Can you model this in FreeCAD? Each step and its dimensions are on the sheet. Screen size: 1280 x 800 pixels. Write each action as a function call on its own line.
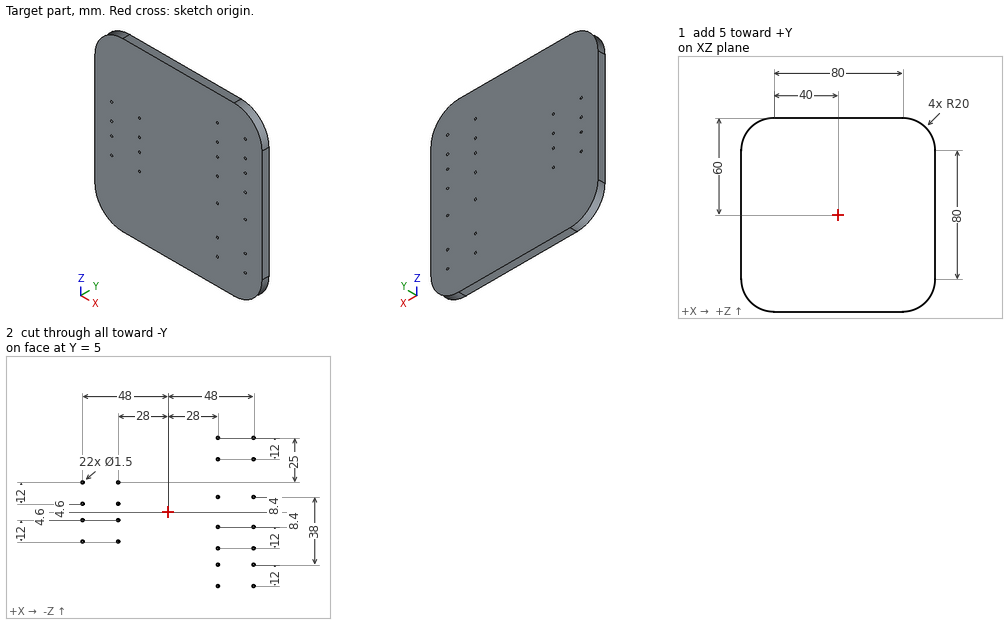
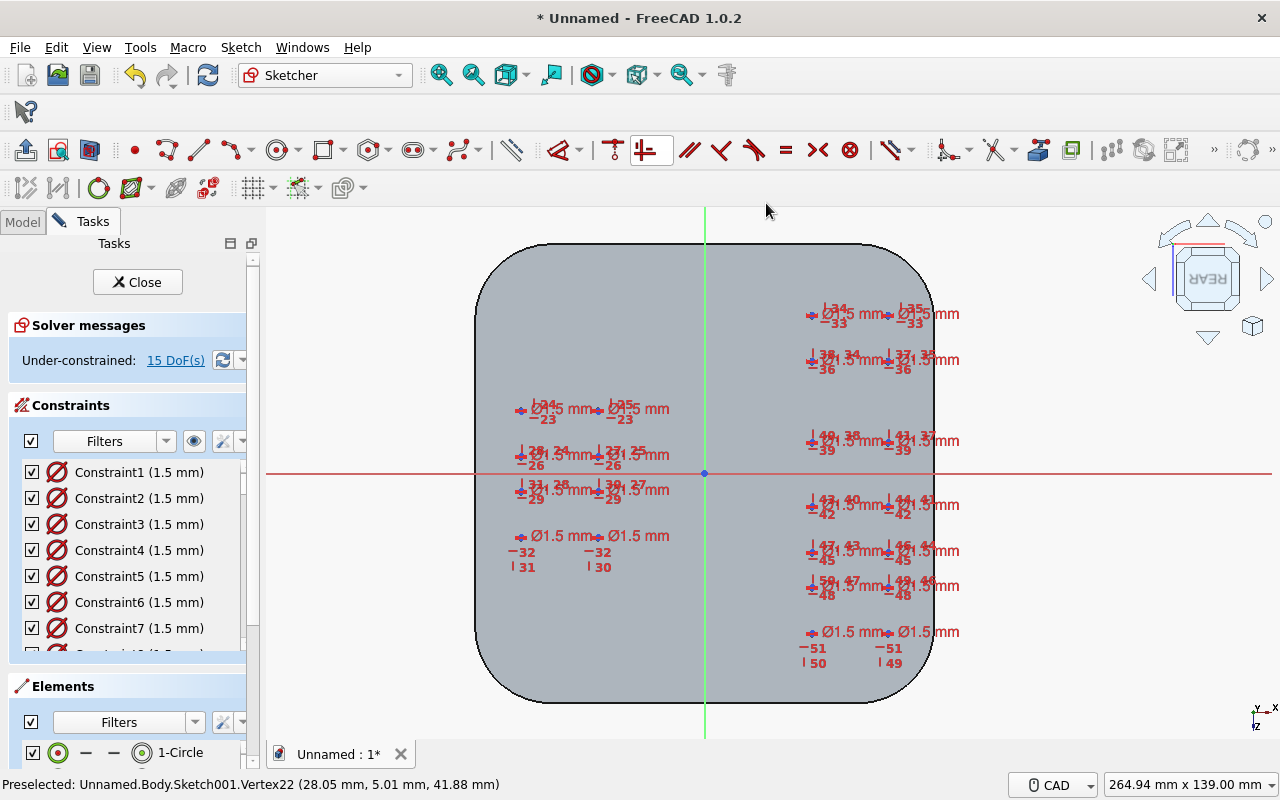
click(558, 150)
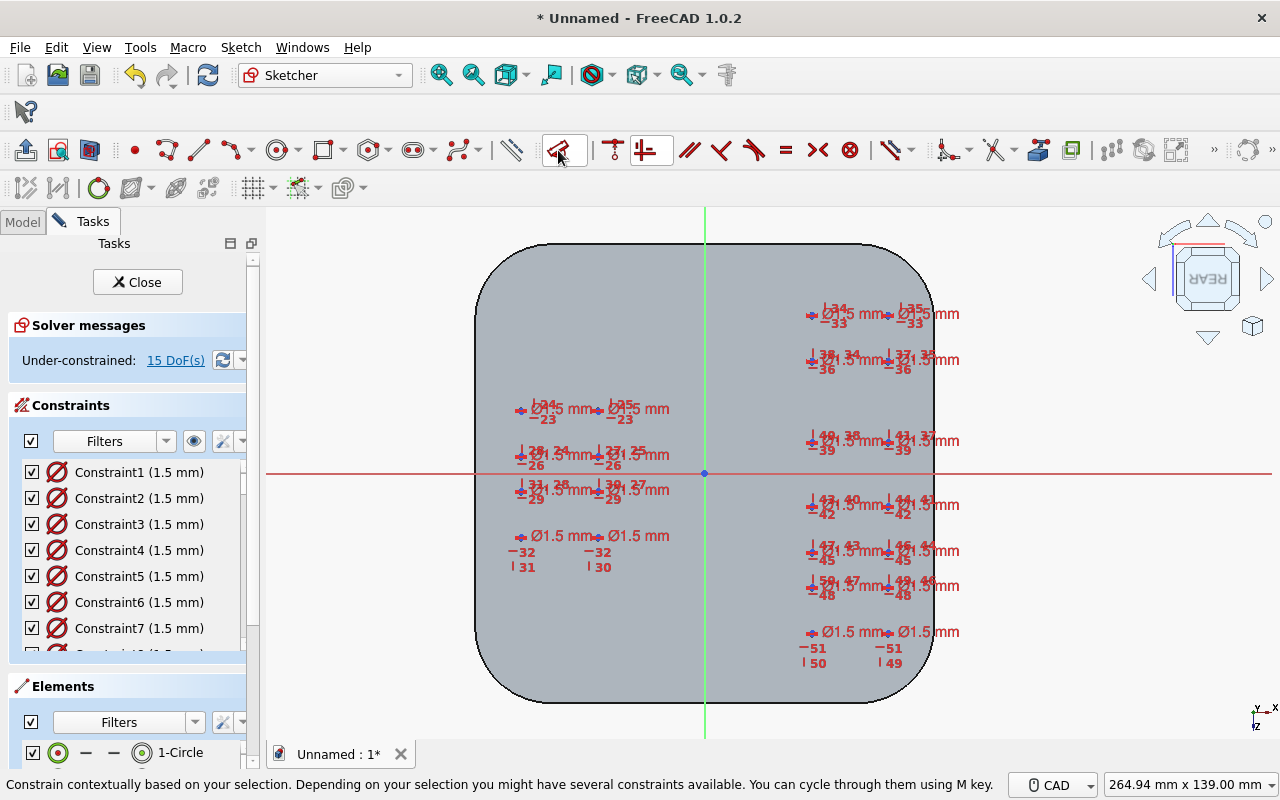
click(521, 411)
click(613, 377)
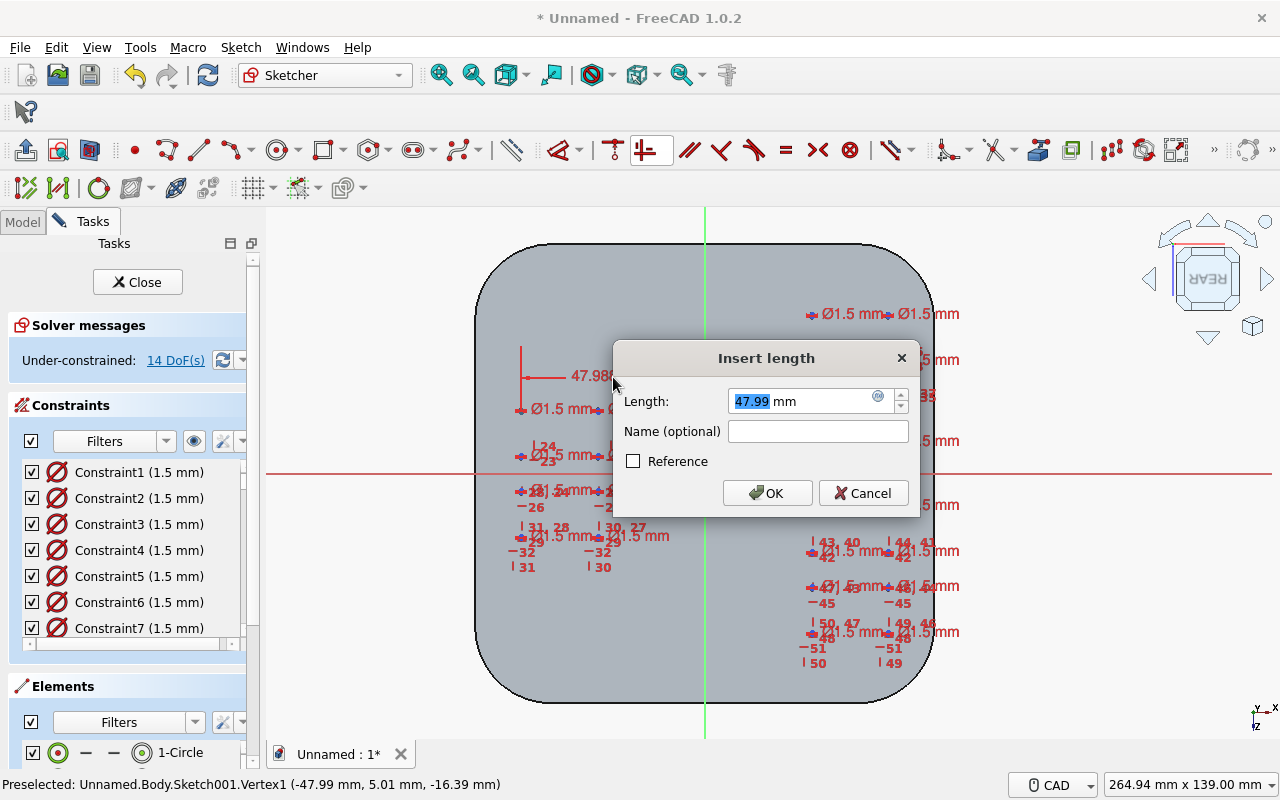
text(48)
key(Return)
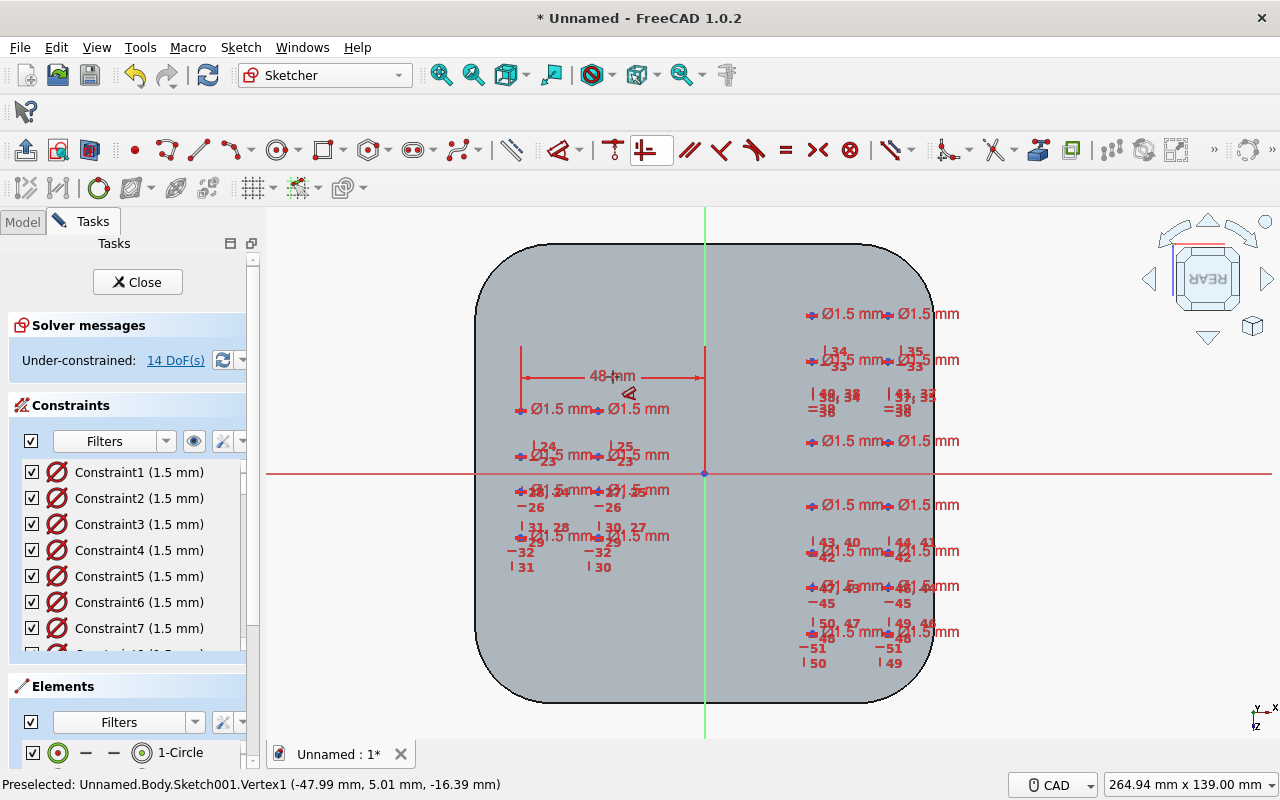
click(598, 411)
click(689, 377)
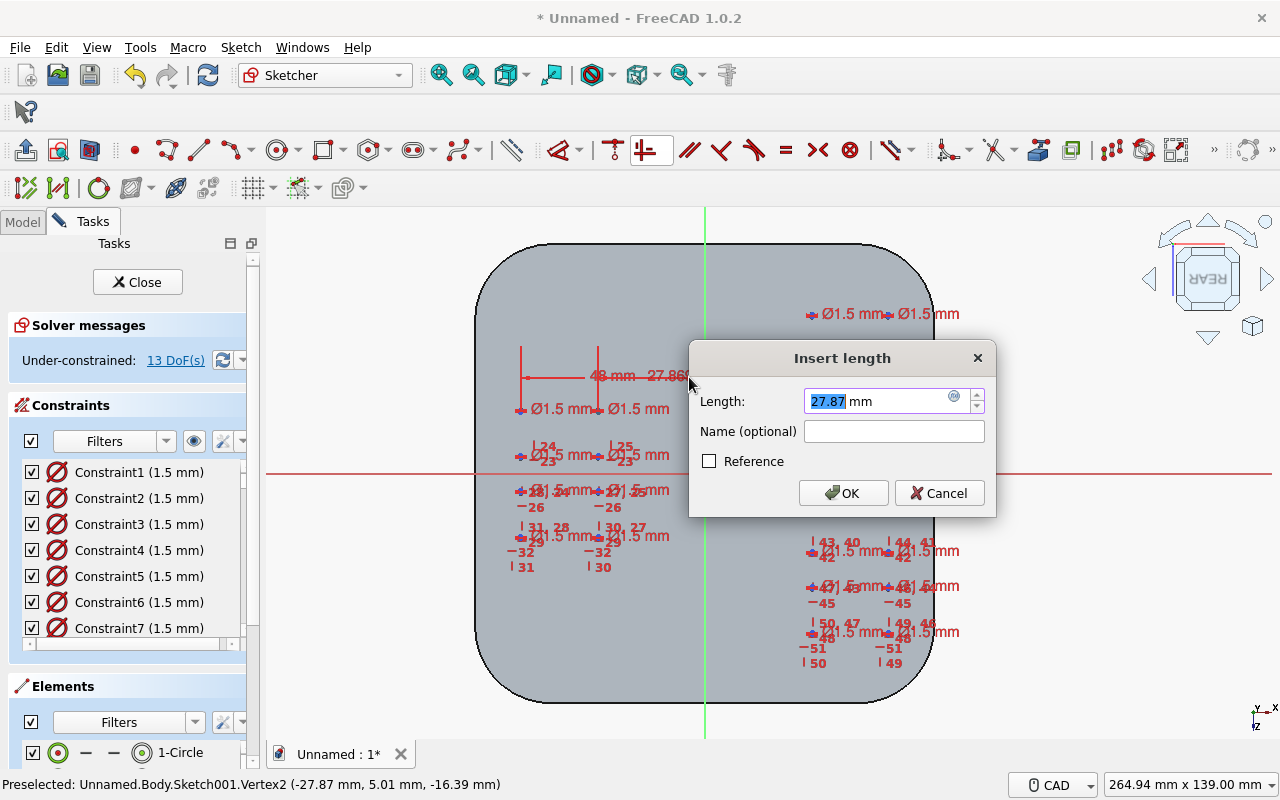
text(28)
key(Return)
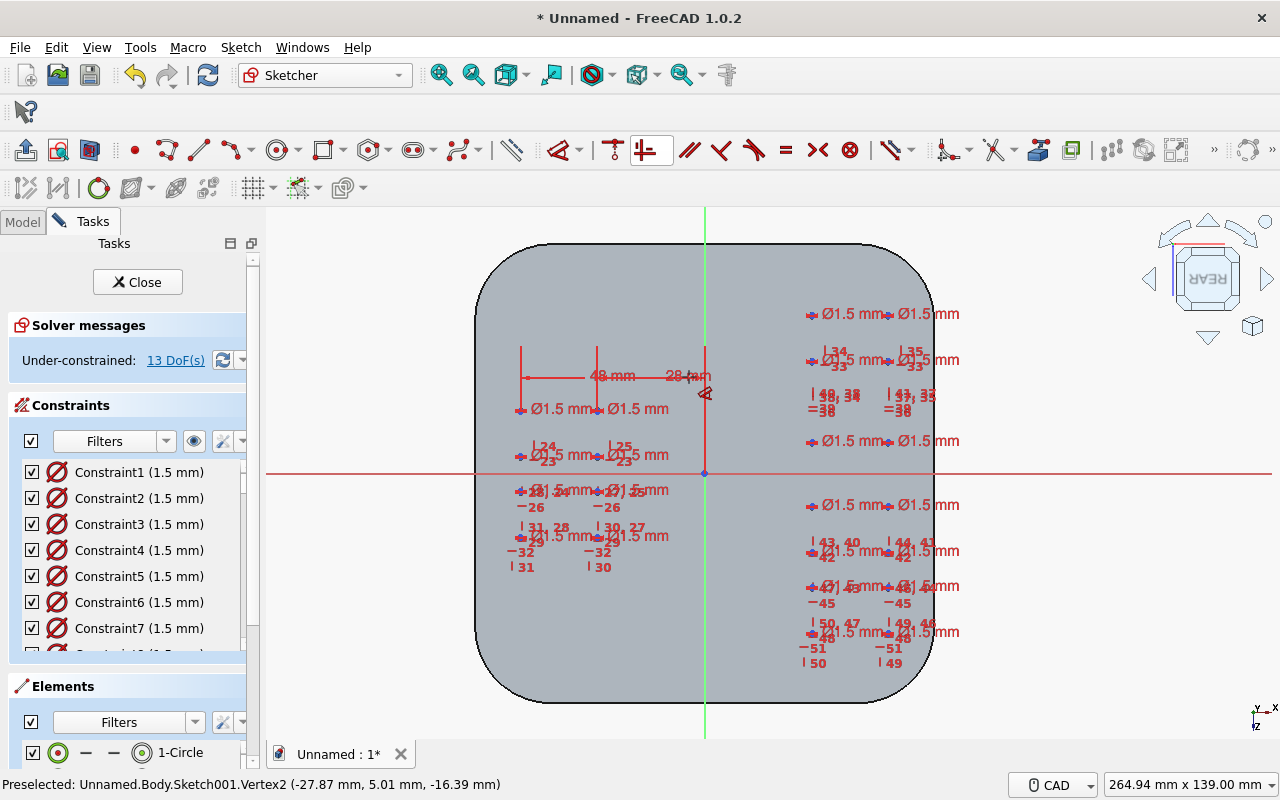
click(812, 316)
click(758, 282)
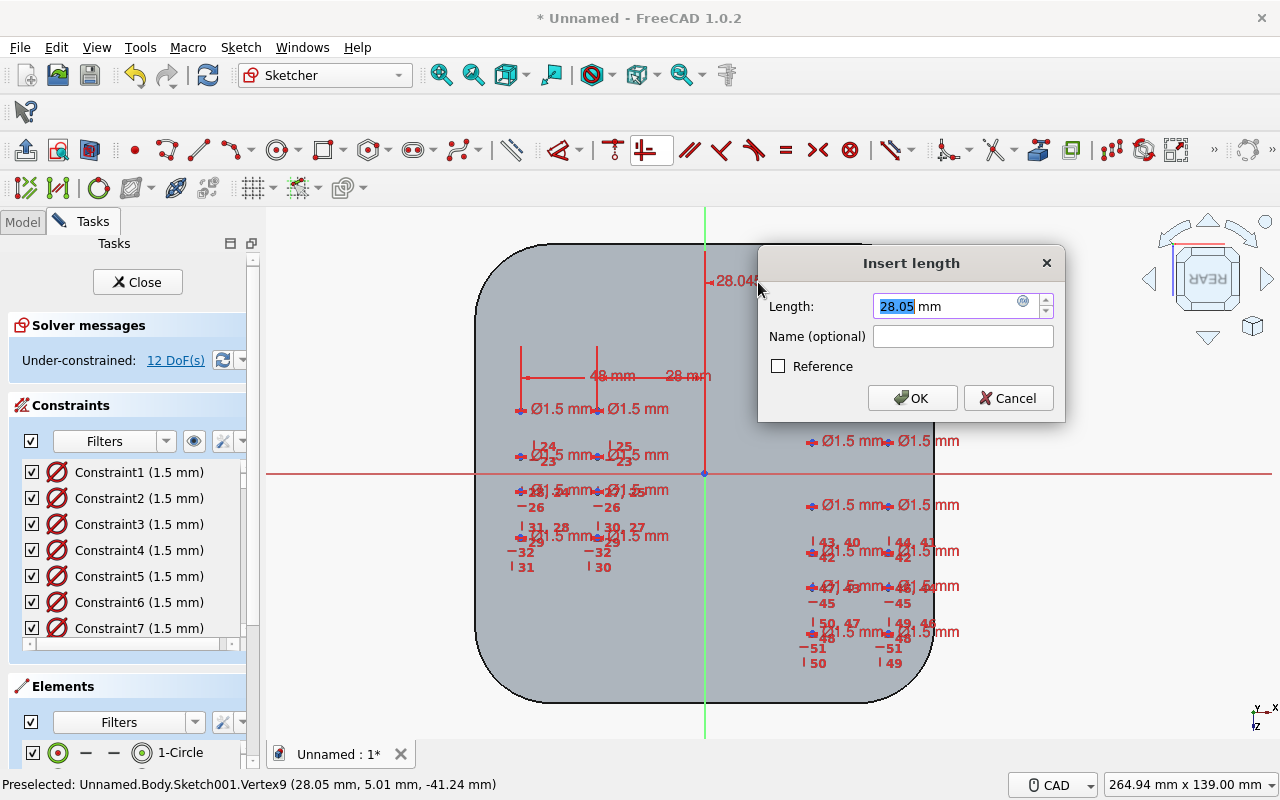
text(28)
key(Return)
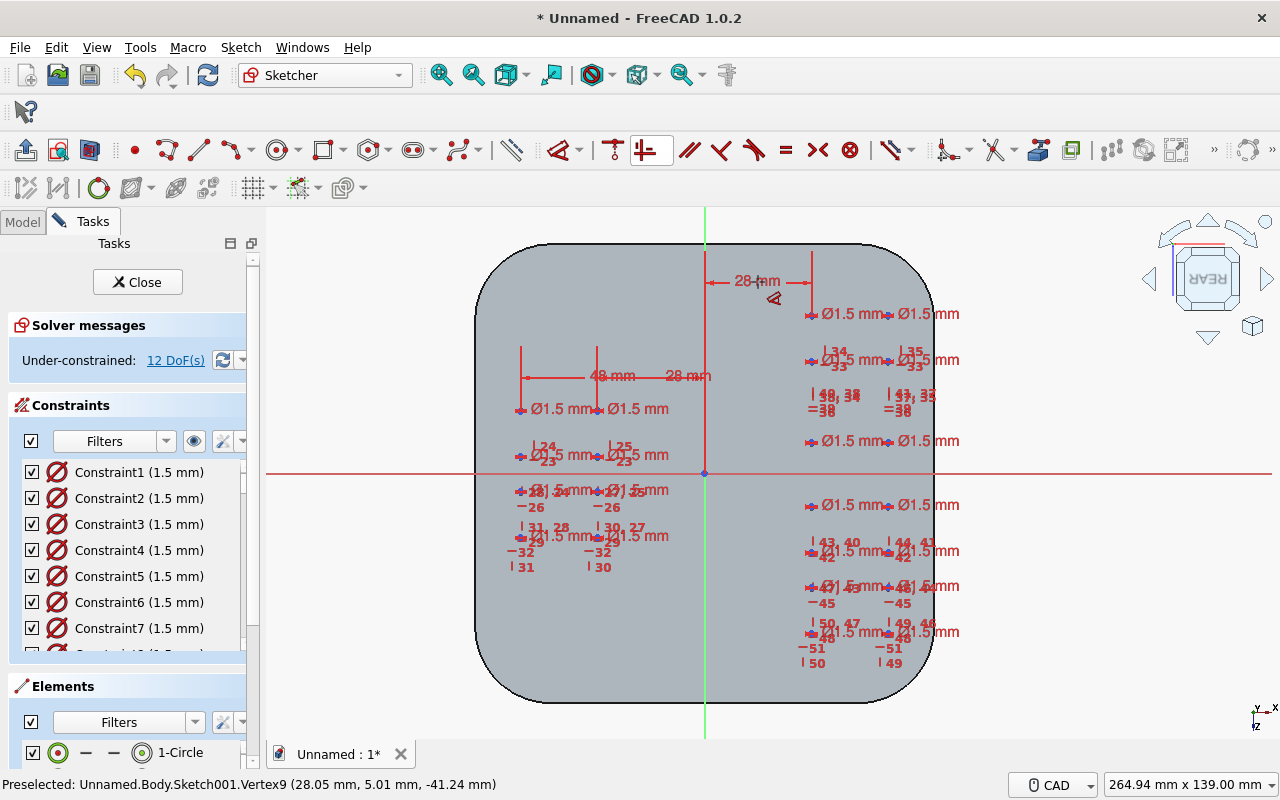
click(888, 316)
click(838, 282)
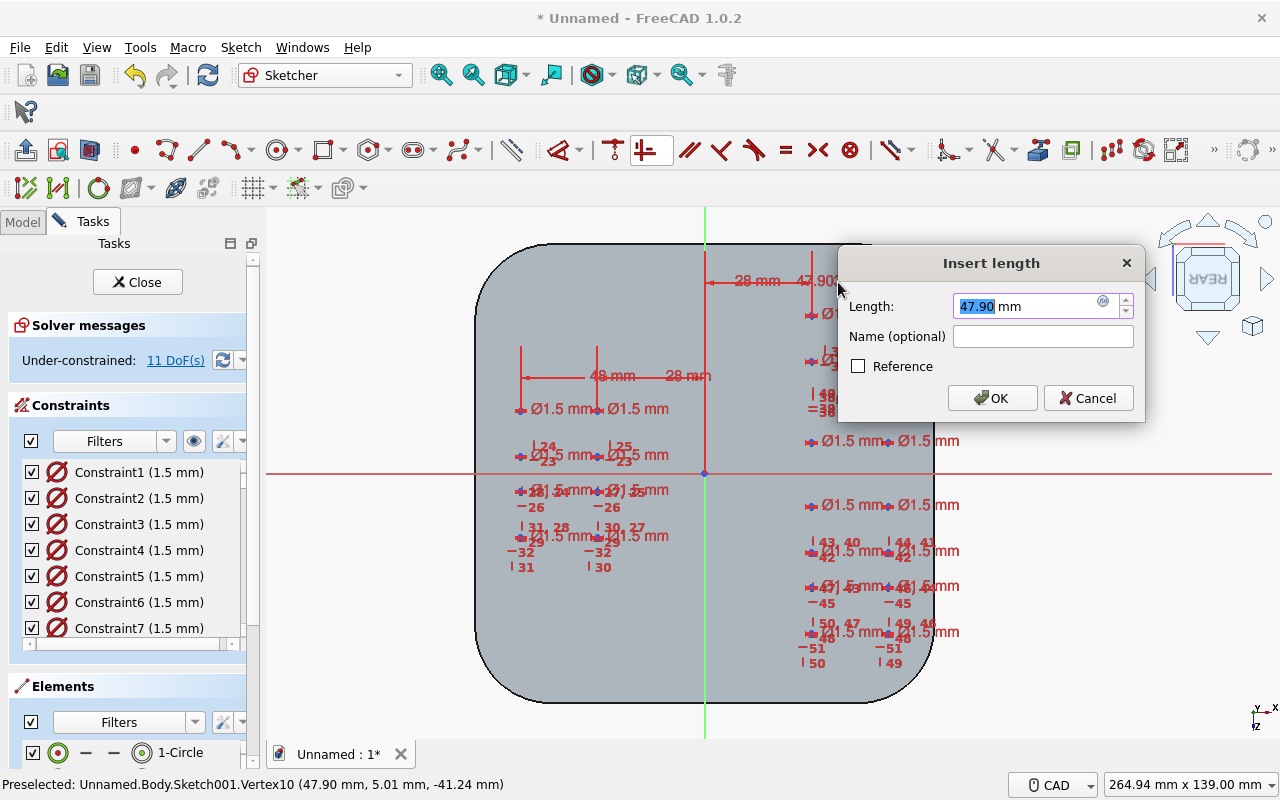
text(48)
key(Return)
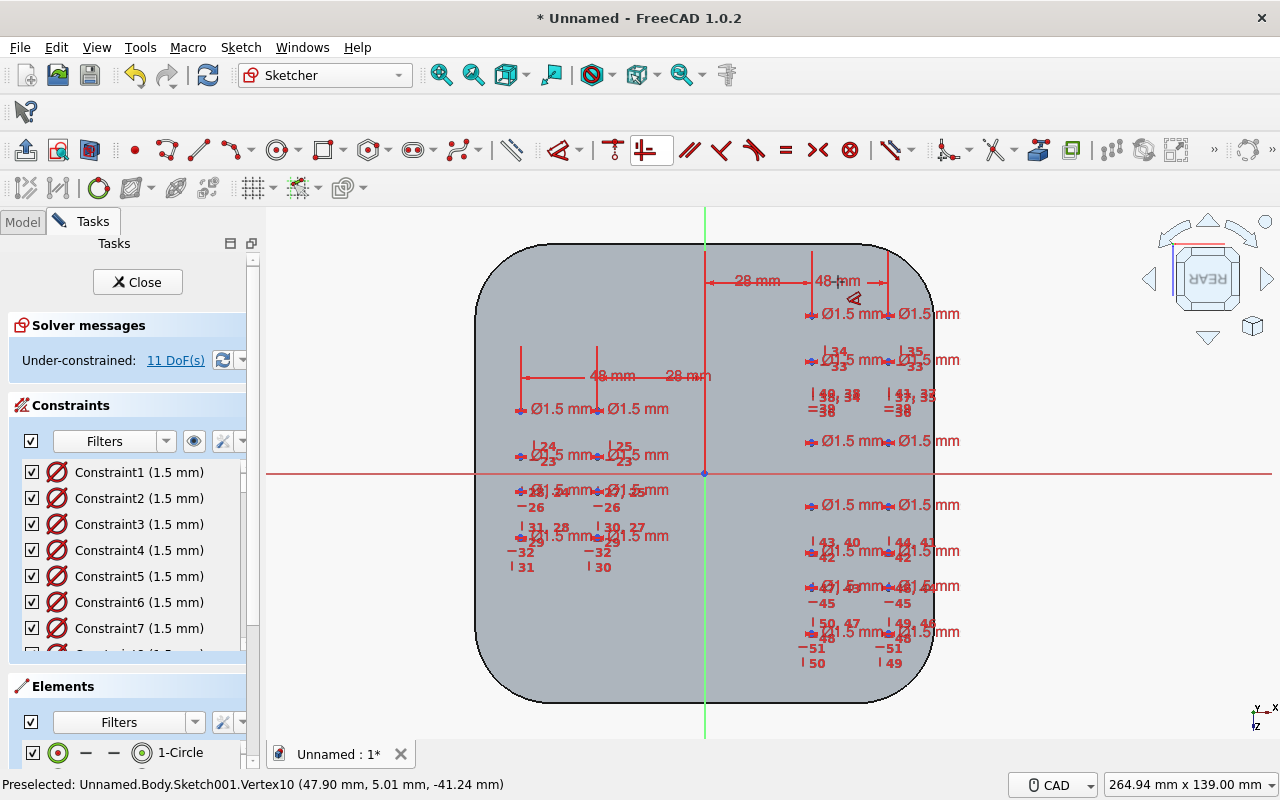
scroll(521, 457, up, 5)